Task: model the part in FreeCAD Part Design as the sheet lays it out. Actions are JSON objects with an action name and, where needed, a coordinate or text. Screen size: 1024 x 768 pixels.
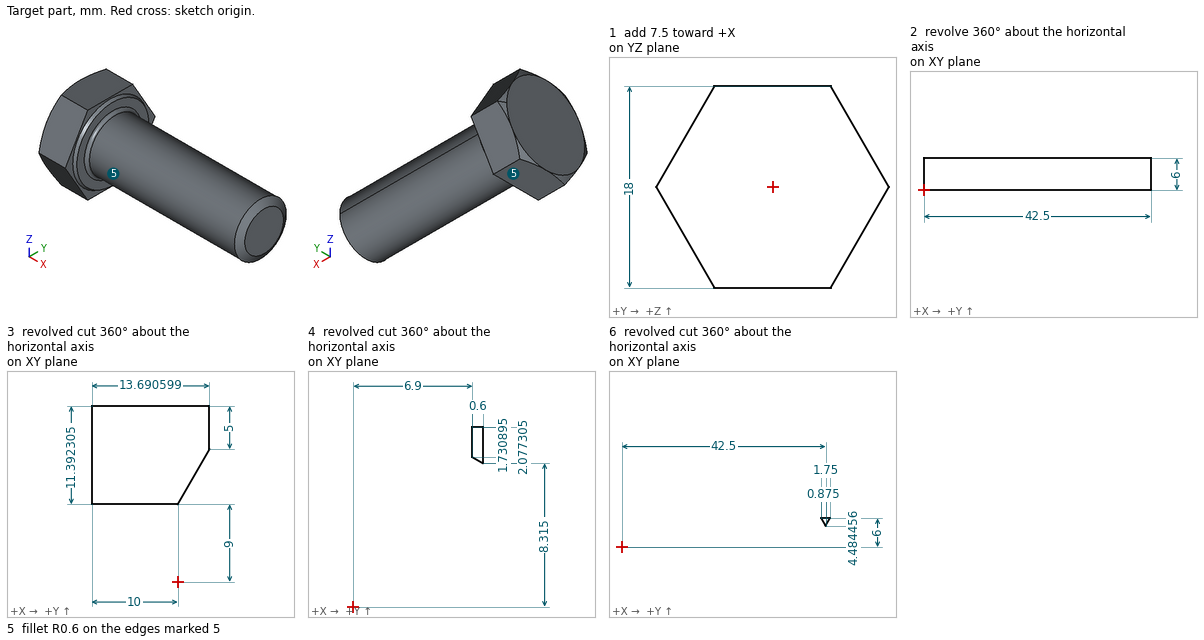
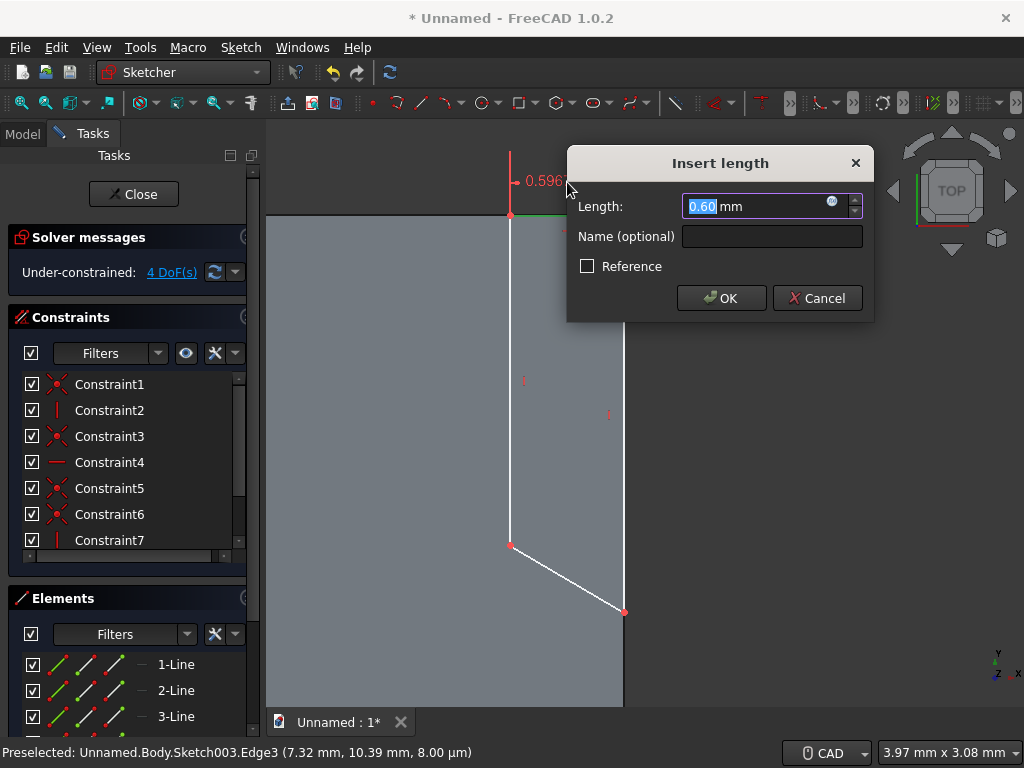
{"action": "type", "text": "0.6"}
{"action": "key", "text": "Return"}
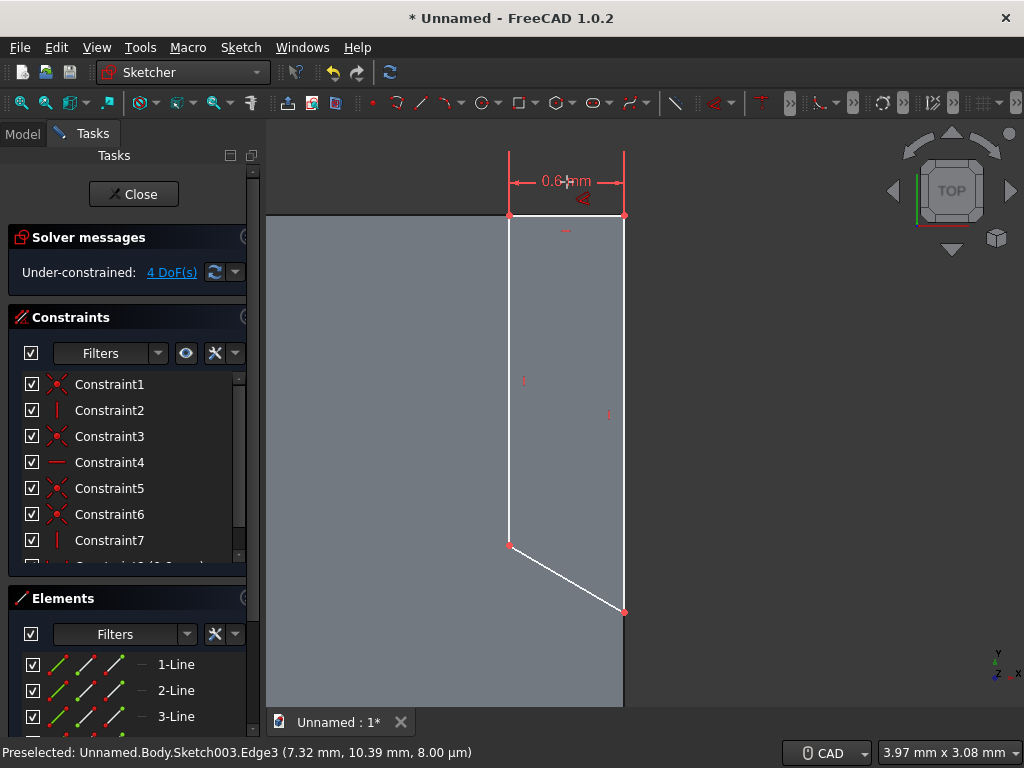
{"action": "left_click", "coordinate": [509, 546]}
{"action": "left_click", "coordinate": [402, 512]}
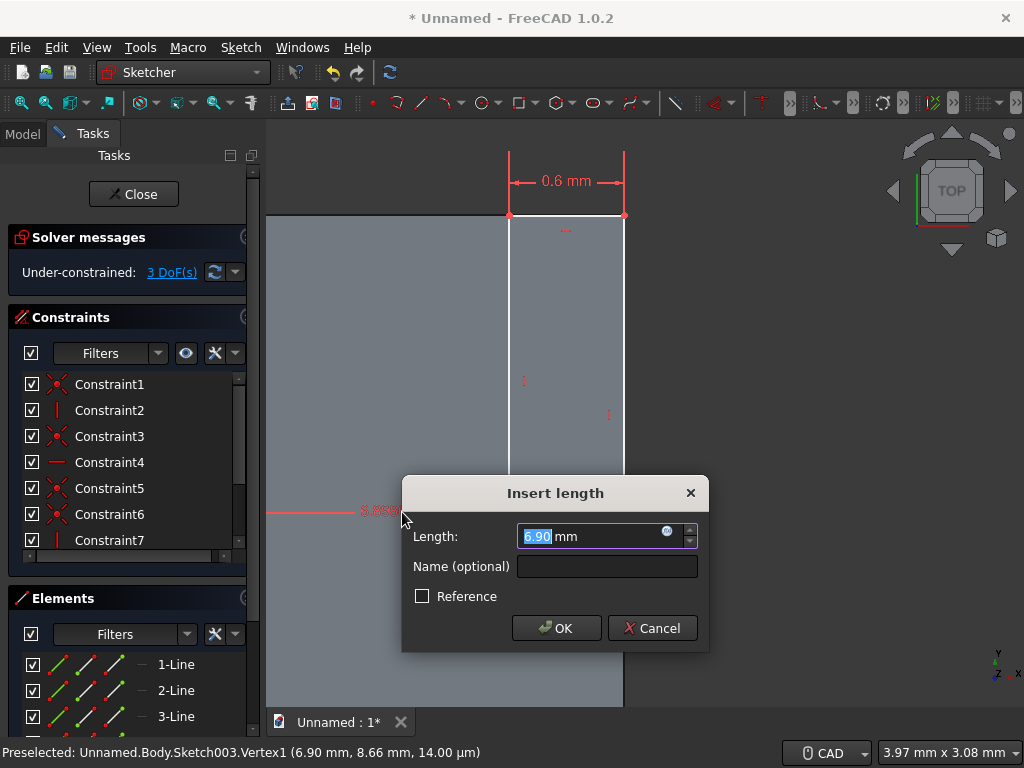
{"action": "type", "text": "6.9"}
{"action": "key", "text": "Return"}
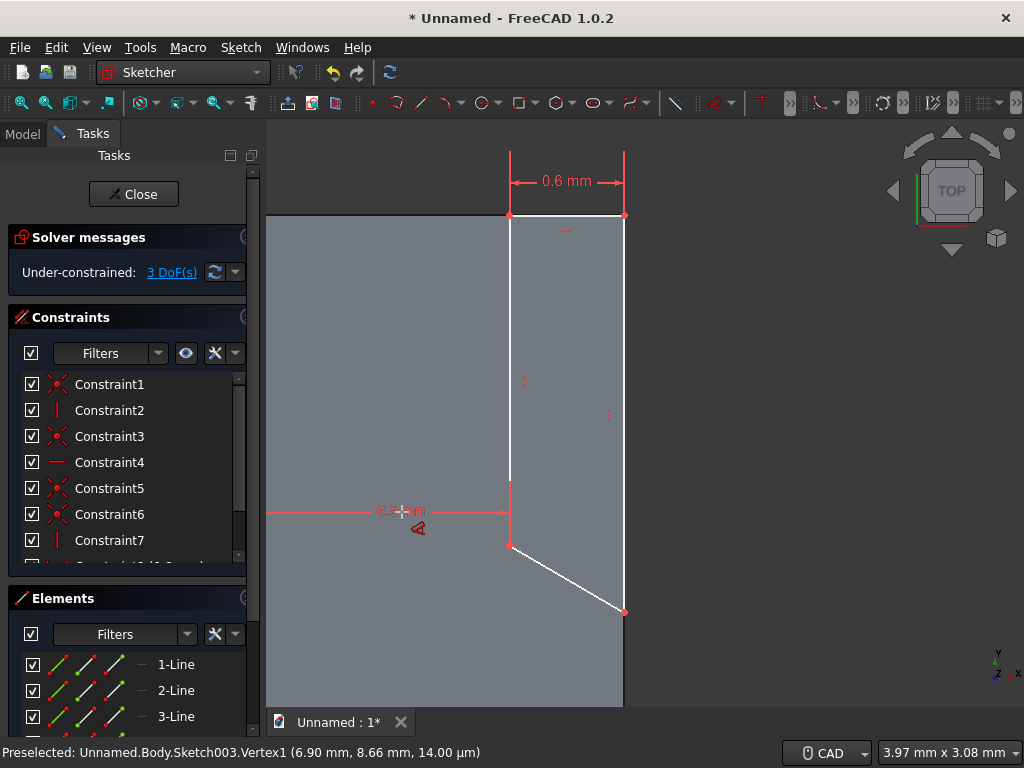
{"action": "left_click", "coordinate": [624, 613]}
{"action": "left_click", "coordinate": [658, 646]}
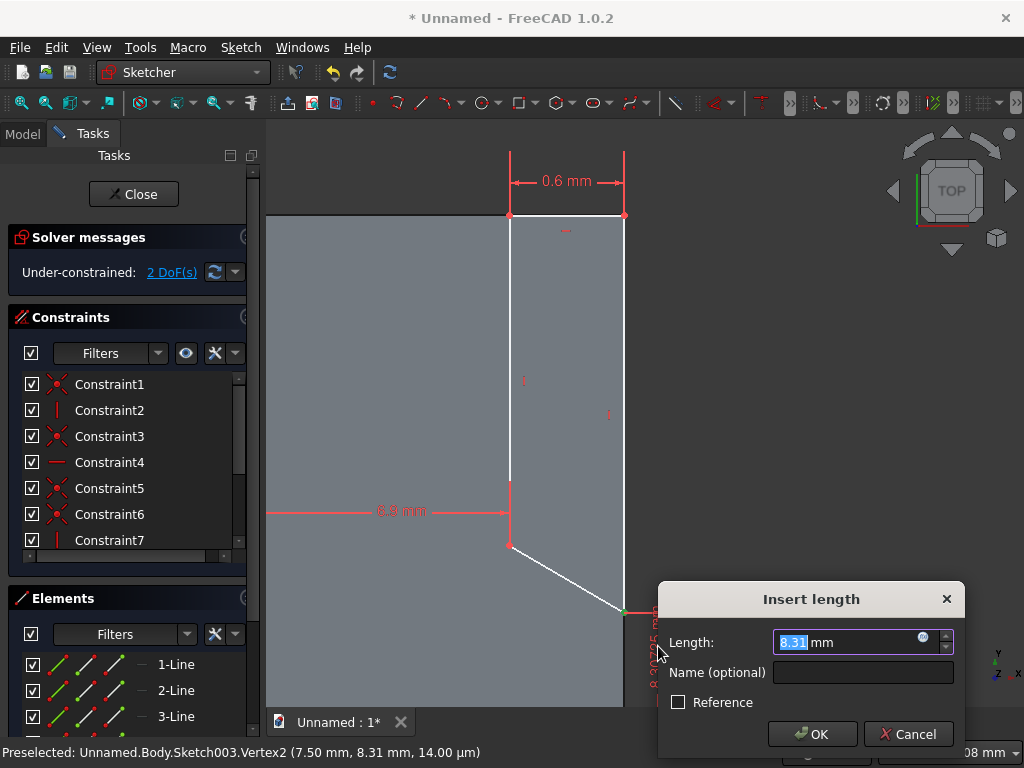
{"action": "type", "text": "8.315"}
{"action": "key", "text": "Return"}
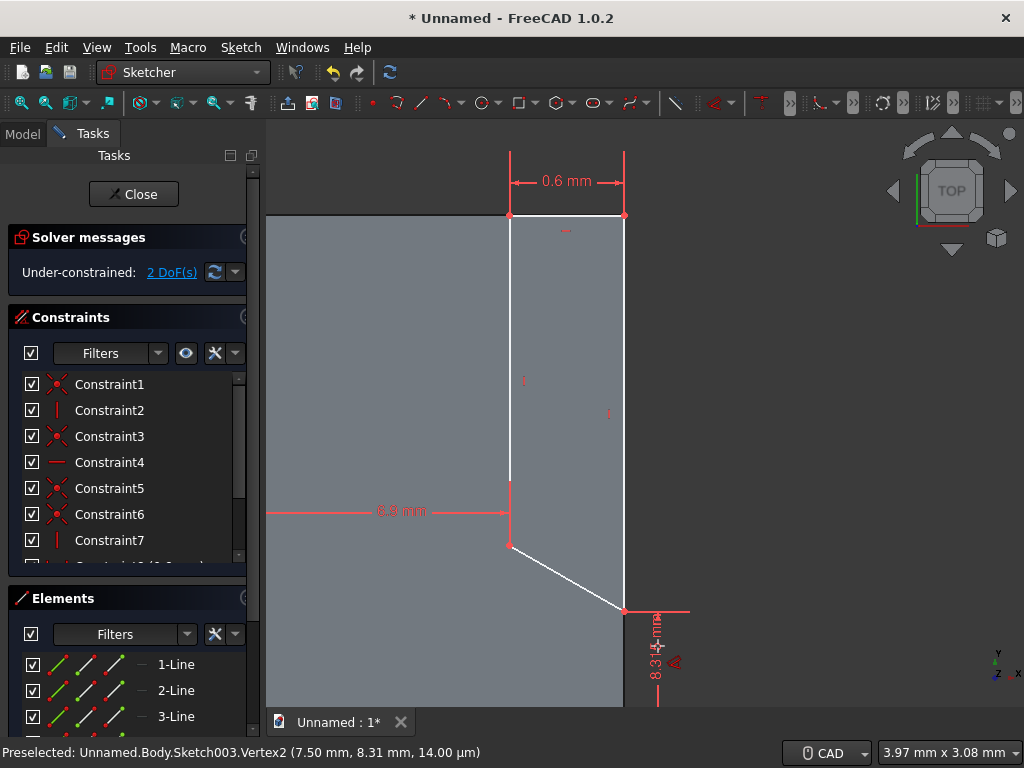
{"action": "left_click", "coordinate": [624, 493]}
{"action": "left_click", "coordinate": [658, 414]}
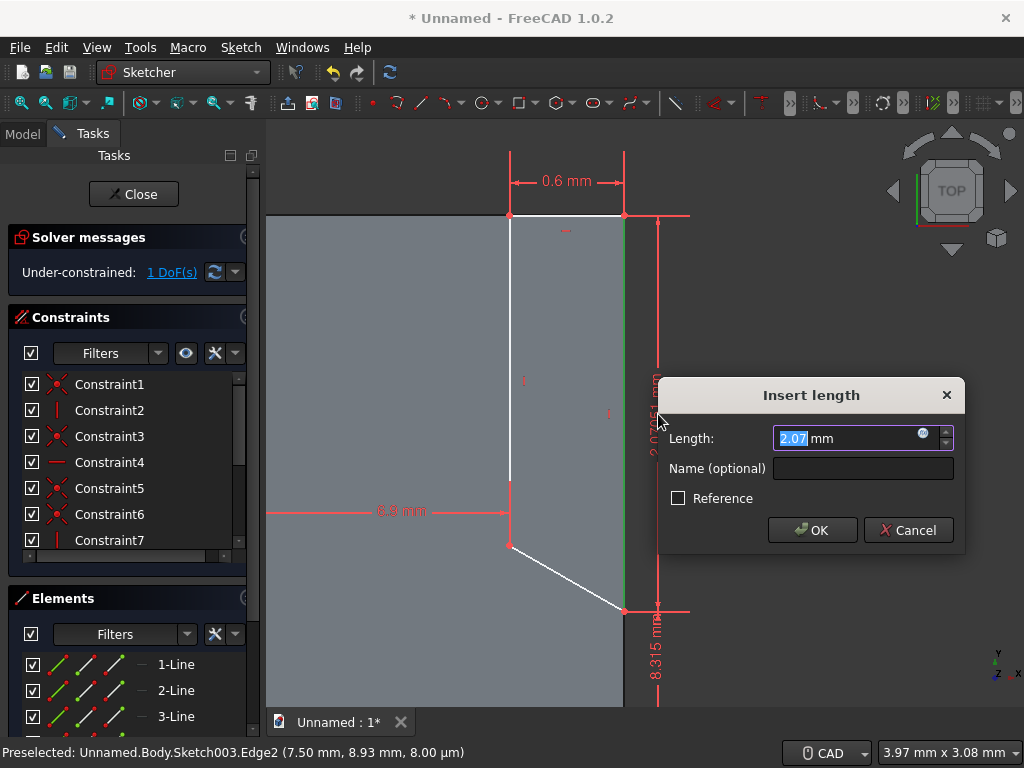
{"action": "type", "text": "2.077305"}
{"action": "key", "text": "Return"}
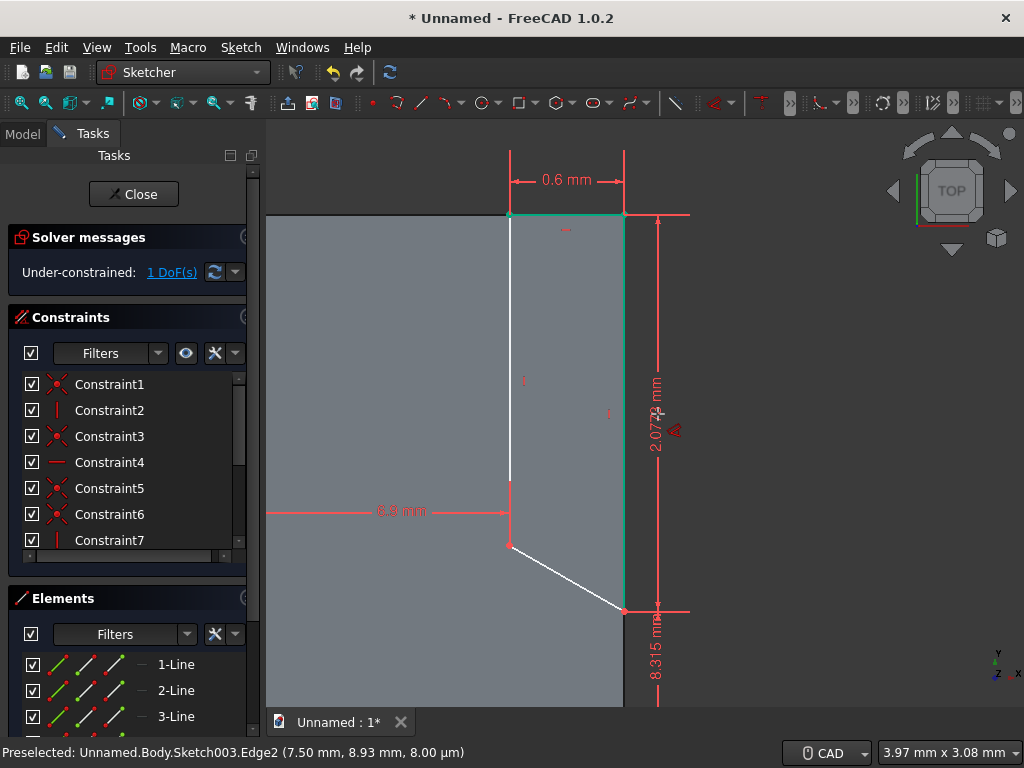
{"action": "left_click", "coordinate": [510, 314]}
{"action": "left_click", "coordinate": [476, 380]}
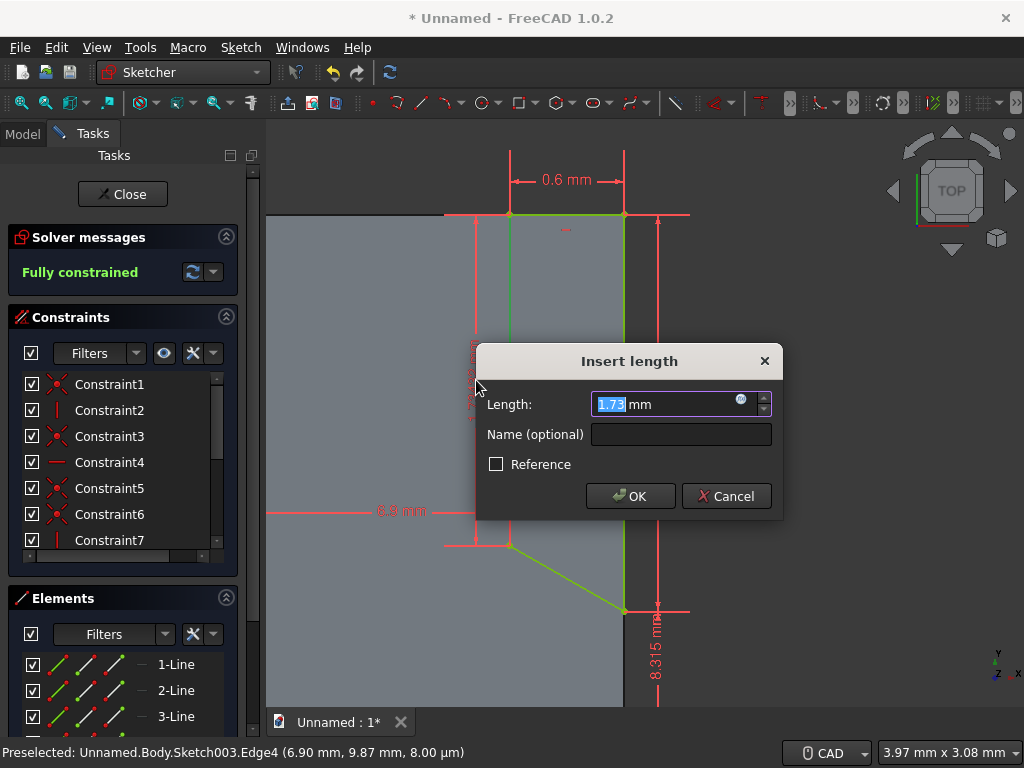
{"action": "type", "text": "1.730895"}
{"action": "key", "text": "Return"}
{"action": "key", "text": "Escape"}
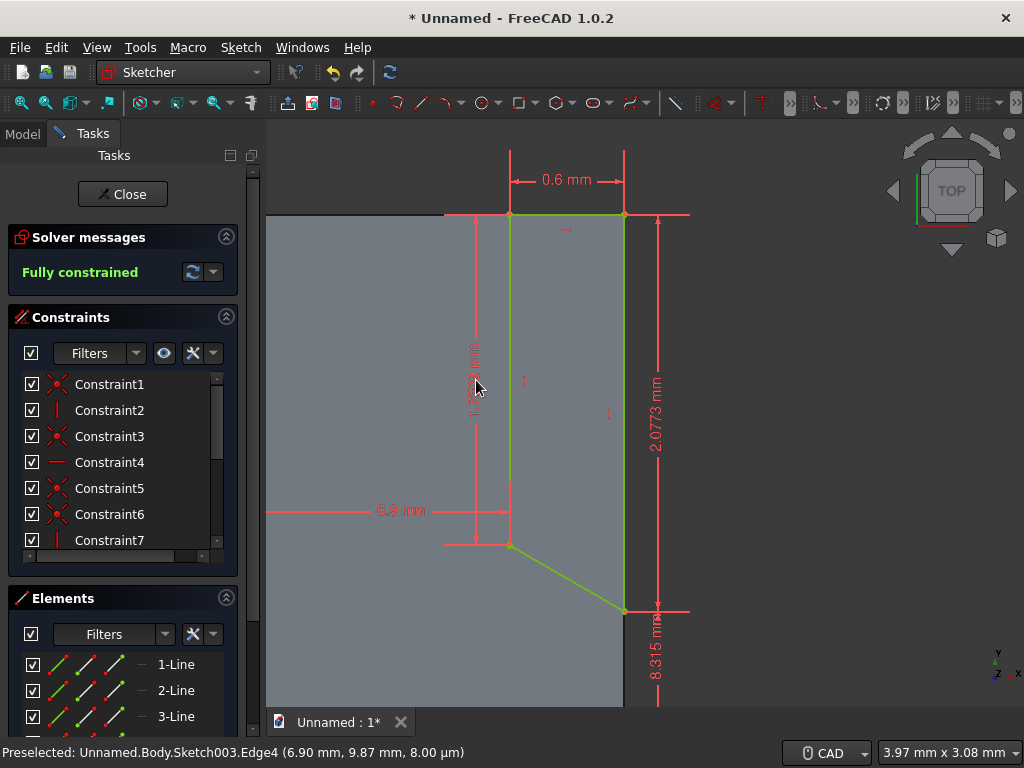
{"action": "left_click", "coordinate": [123, 194]}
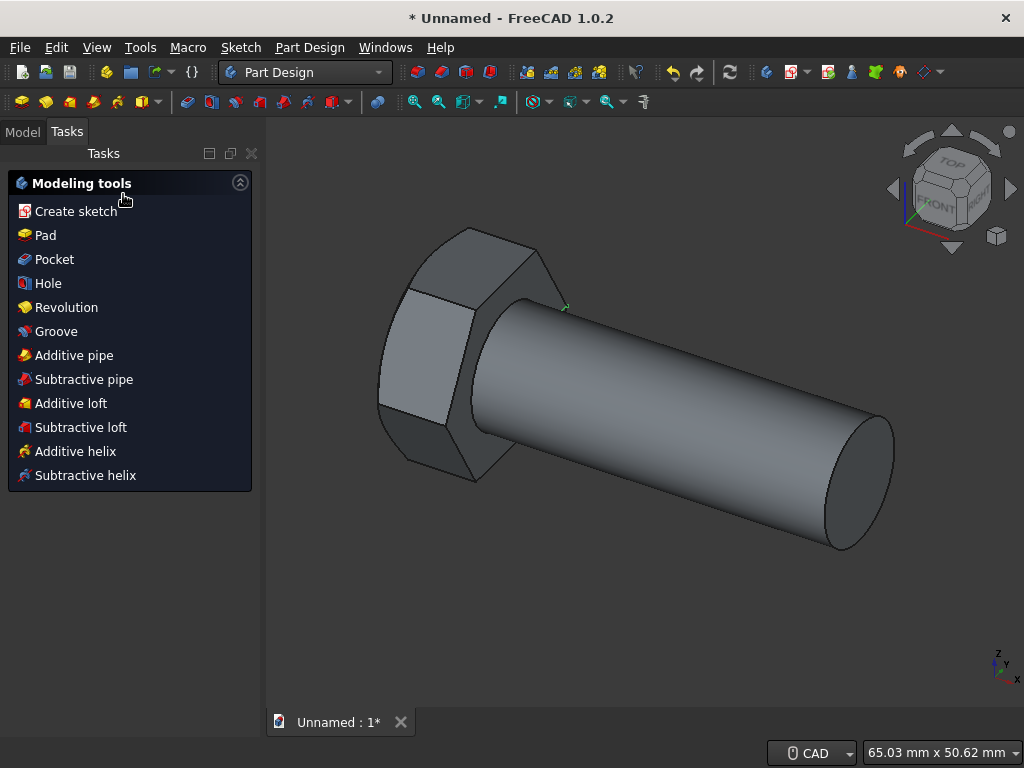
{"action": "left_click", "coordinate": [236, 102]}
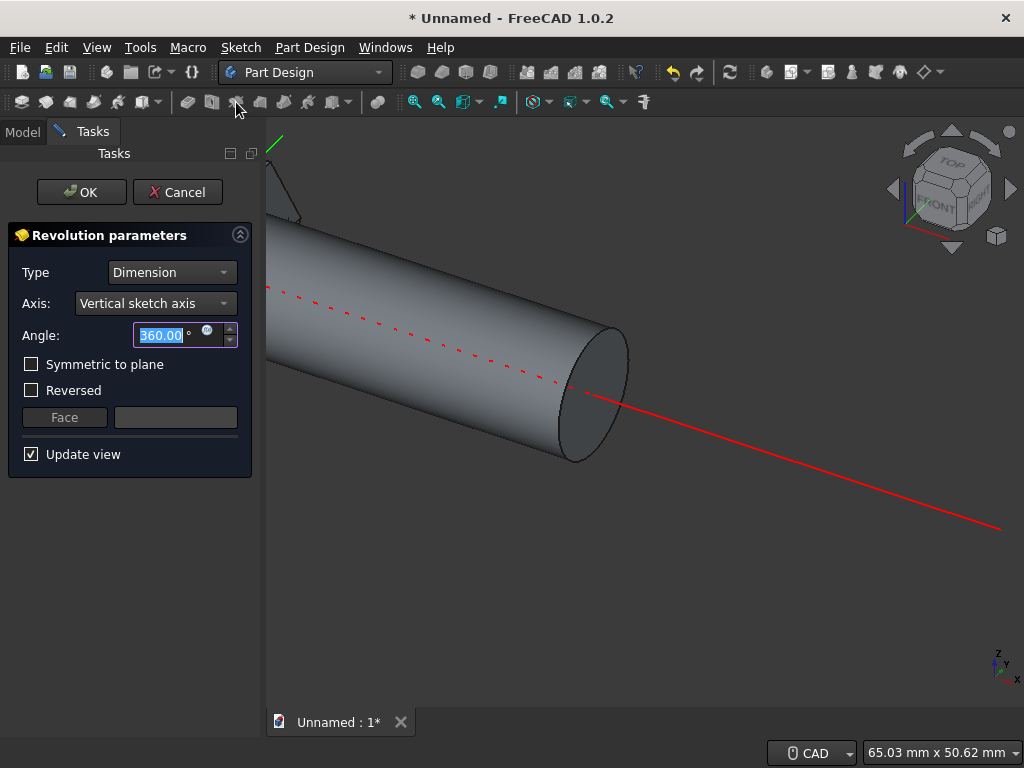
{"action": "left_click", "coordinate": [156, 304]}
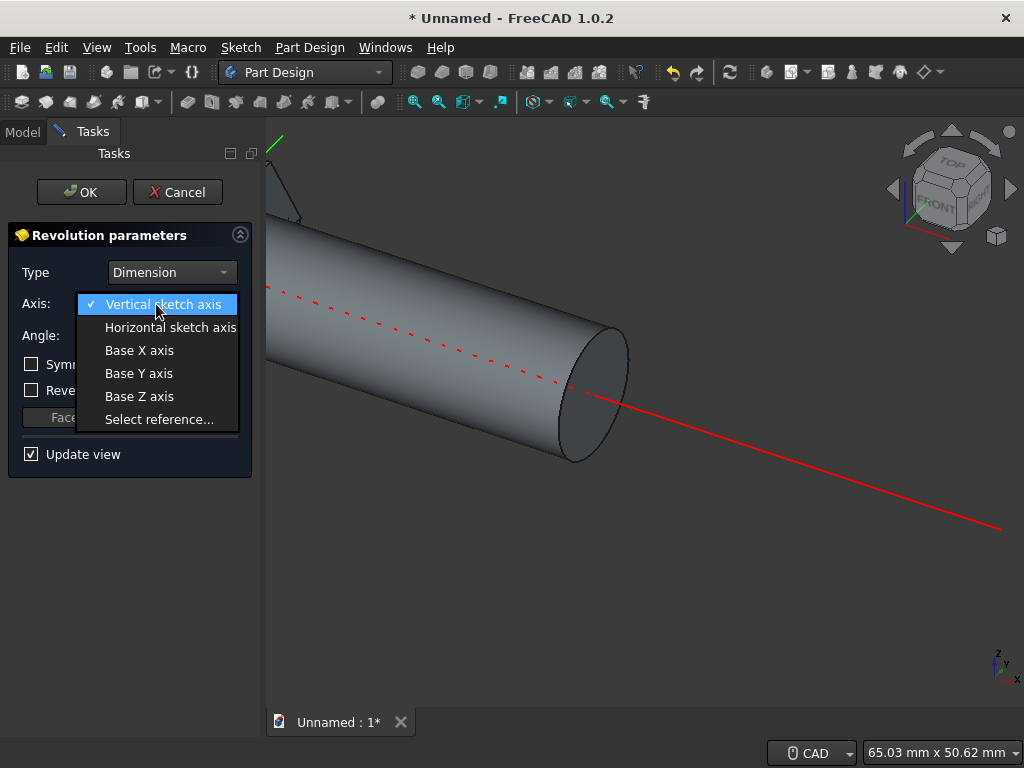
{"action": "left_click", "coordinate": [156, 328]}